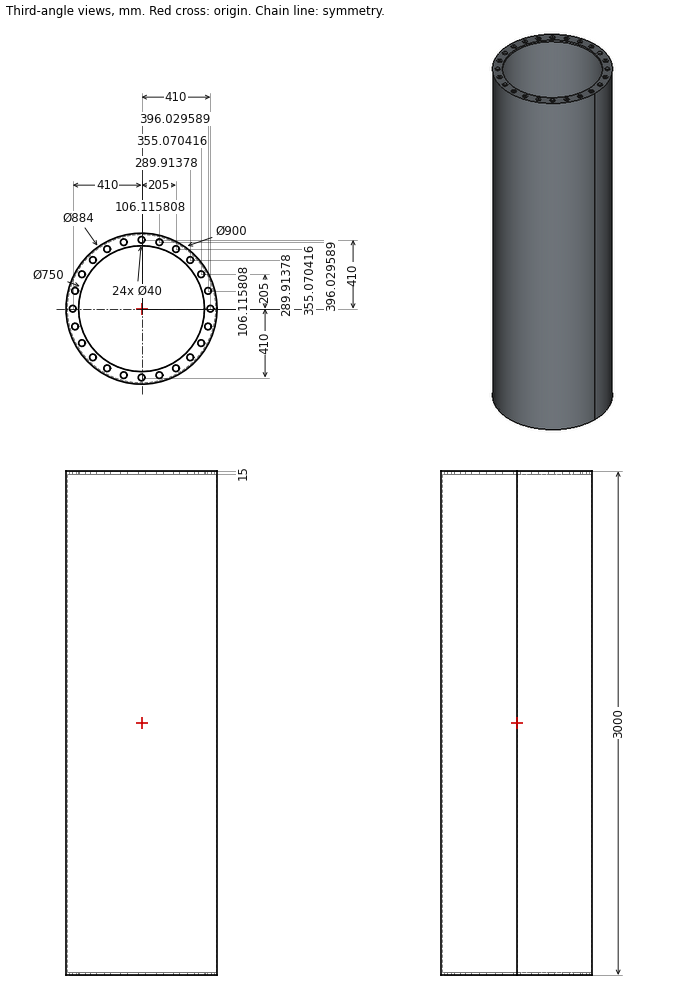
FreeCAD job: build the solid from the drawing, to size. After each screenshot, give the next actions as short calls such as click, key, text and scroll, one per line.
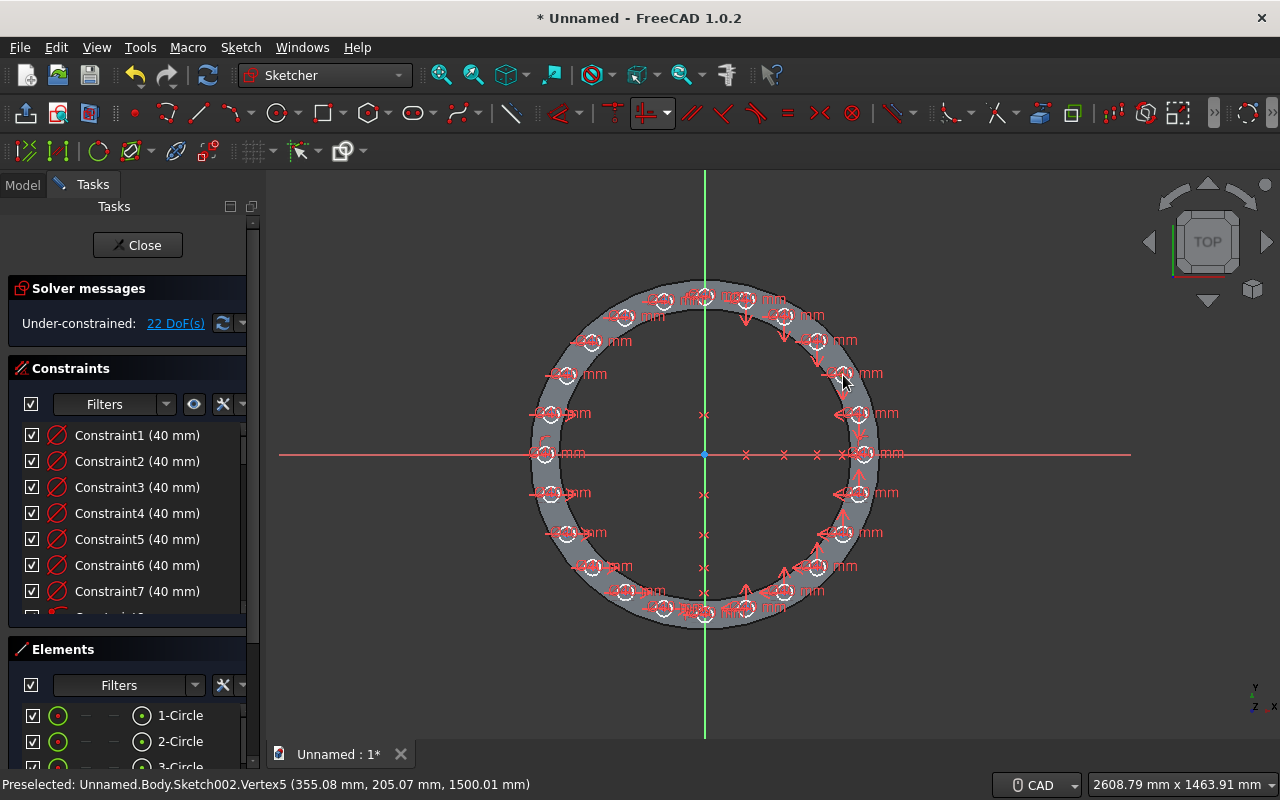
click(567, 376)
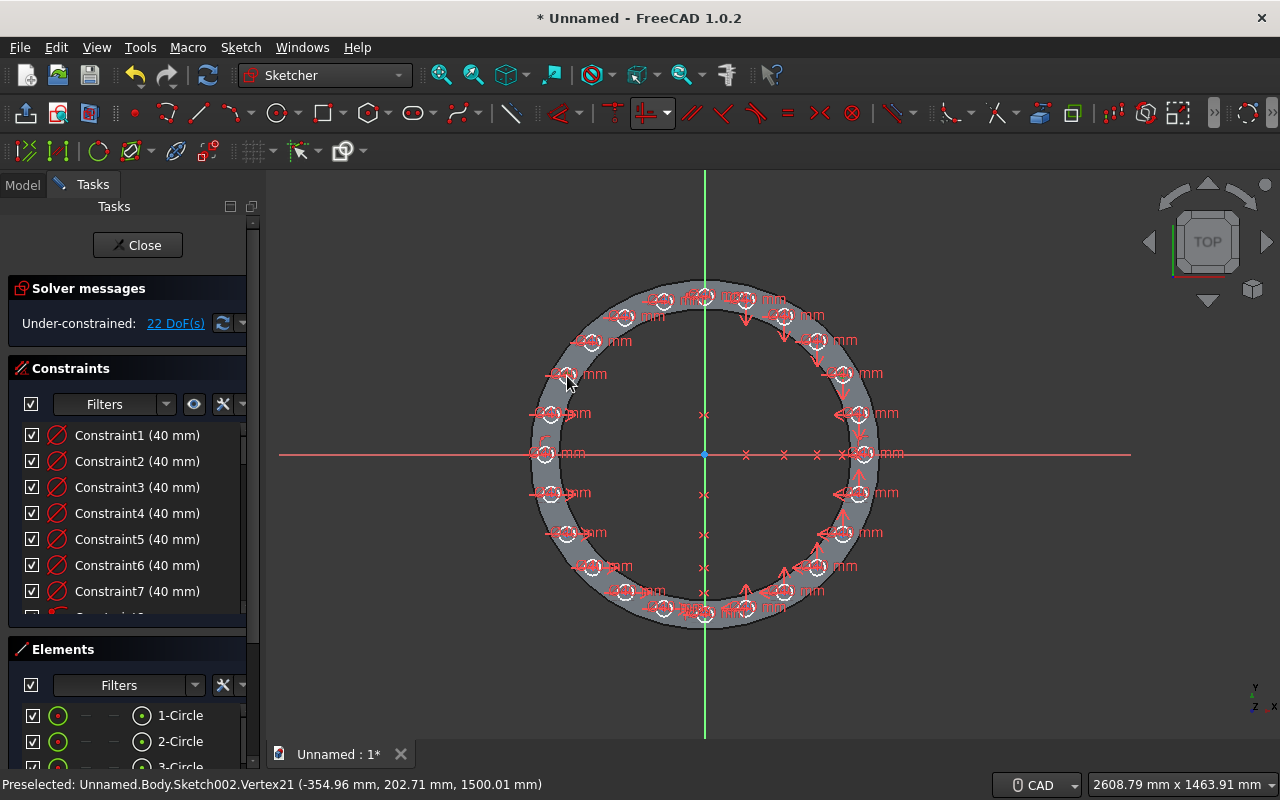
click(705, 674)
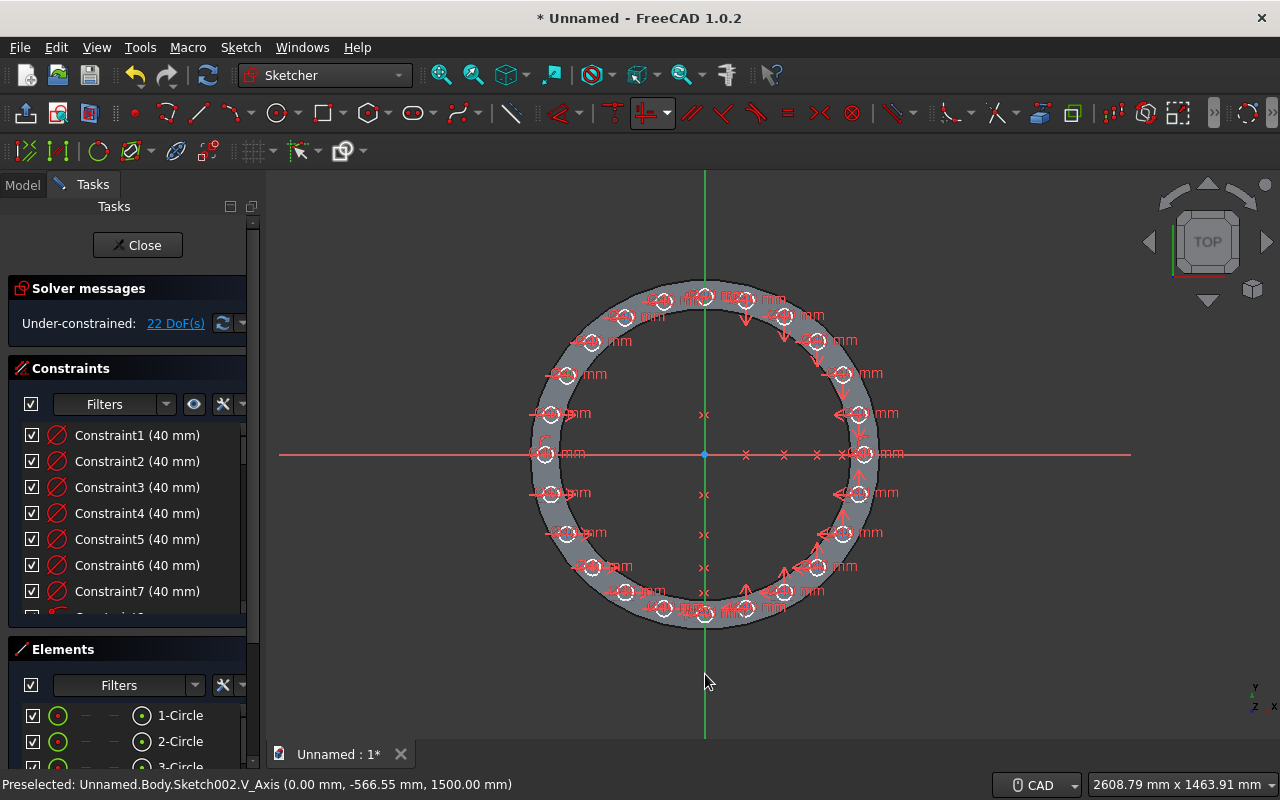
click(820, 114)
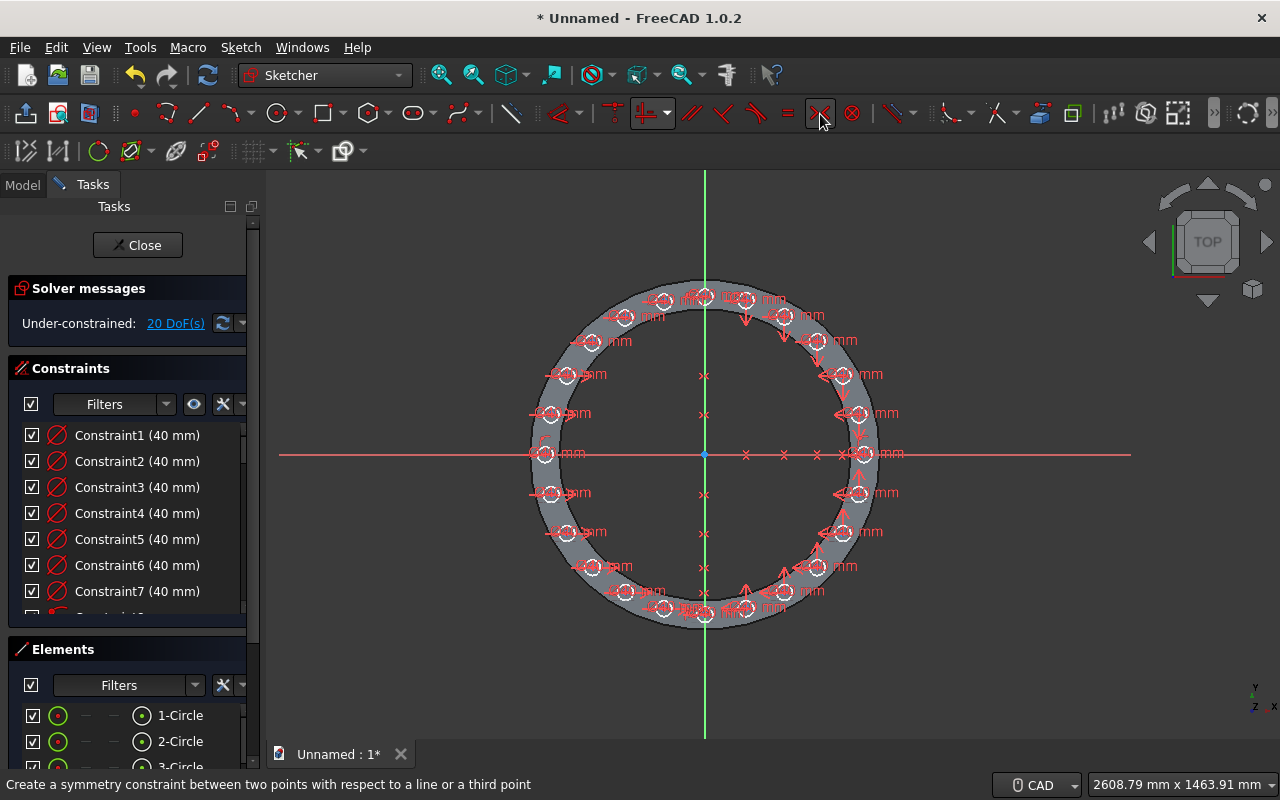
click(817, 342)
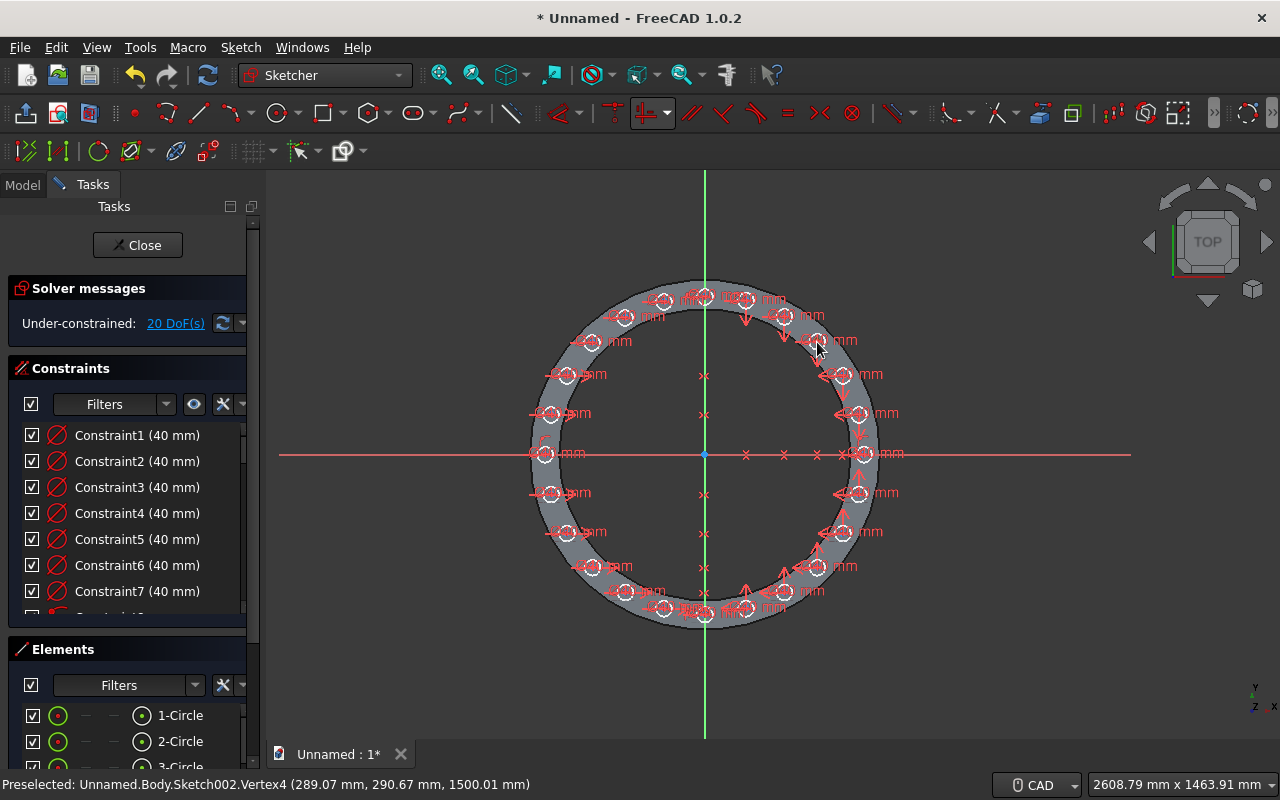
click(592, 343)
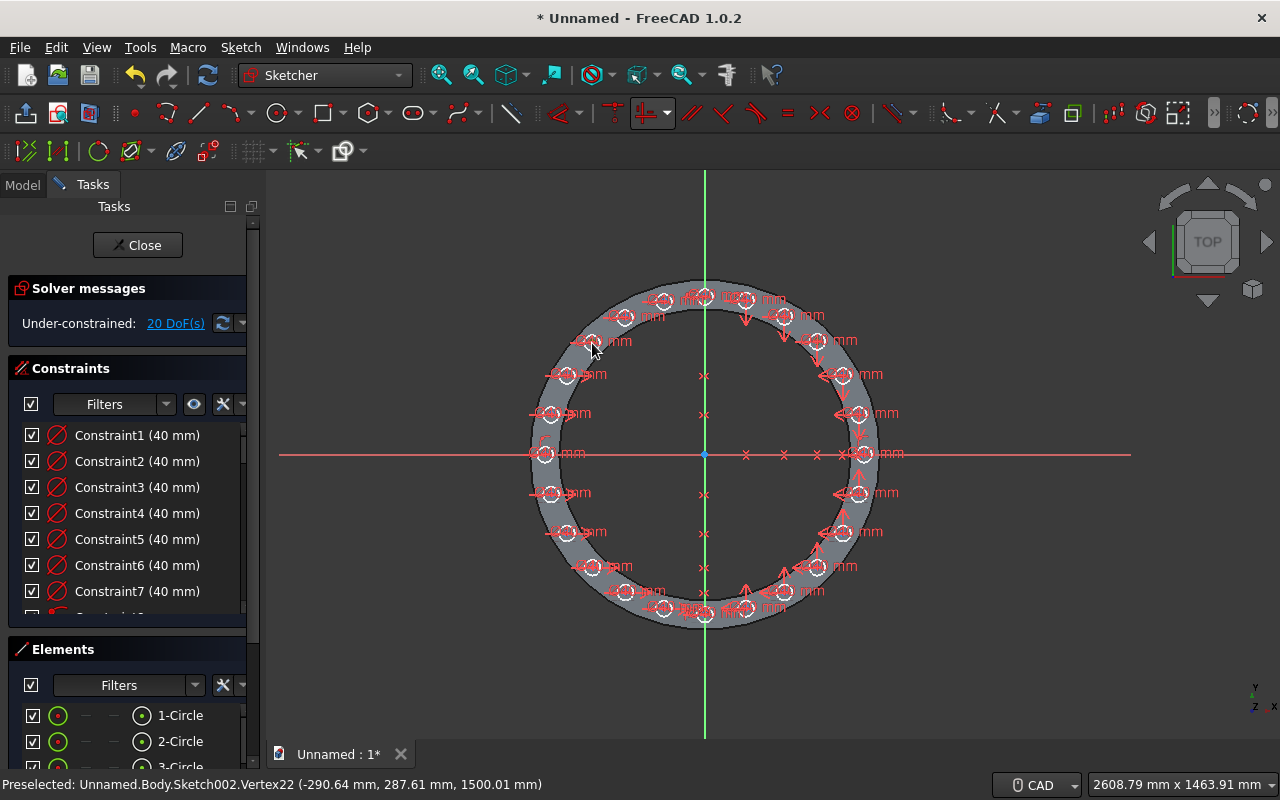
click(705, 674)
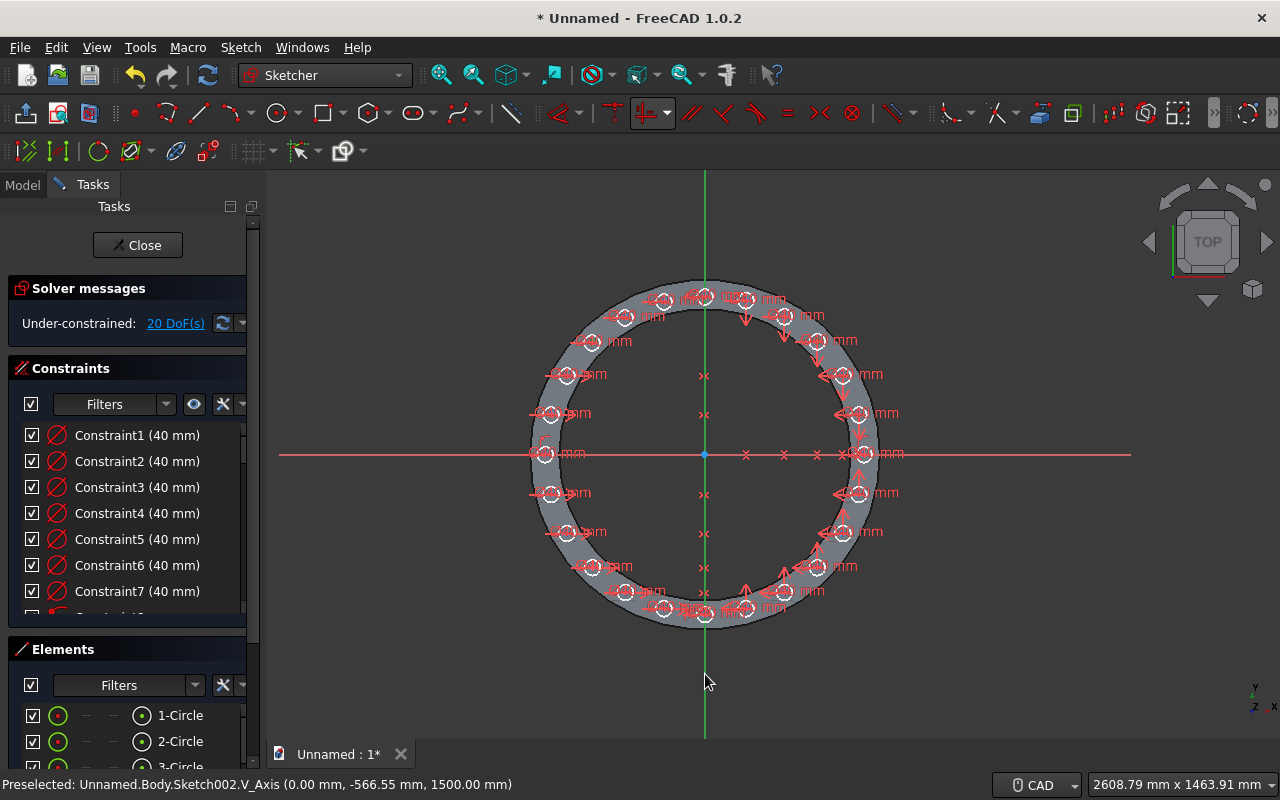
click(820, 114)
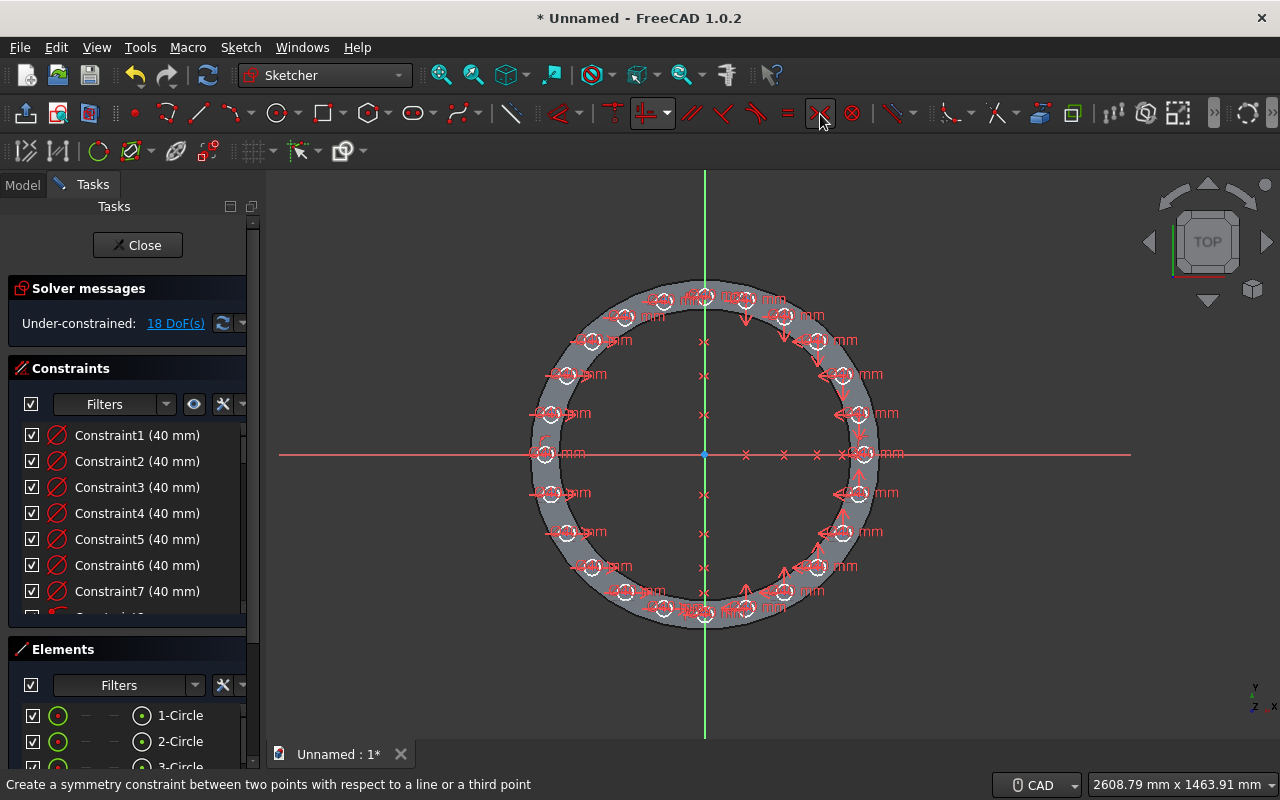
click(784, 317)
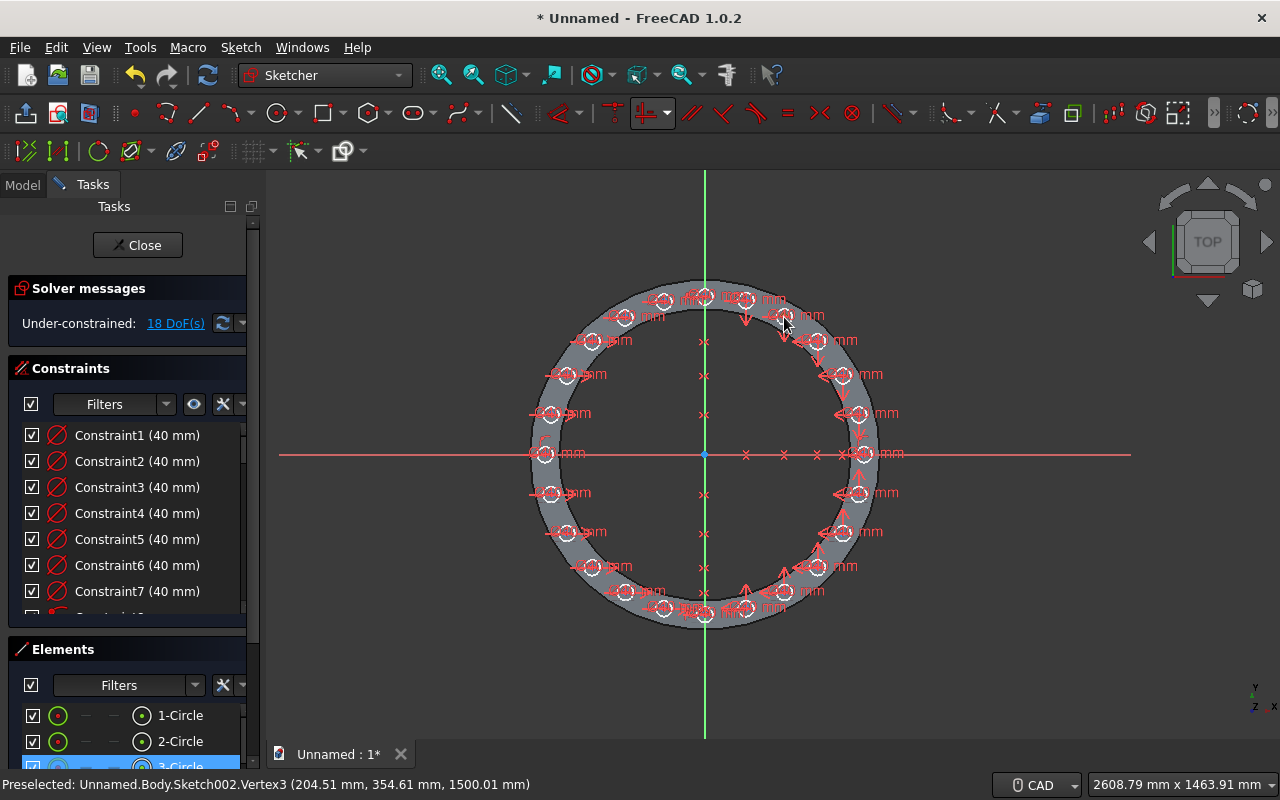
click(625, 318)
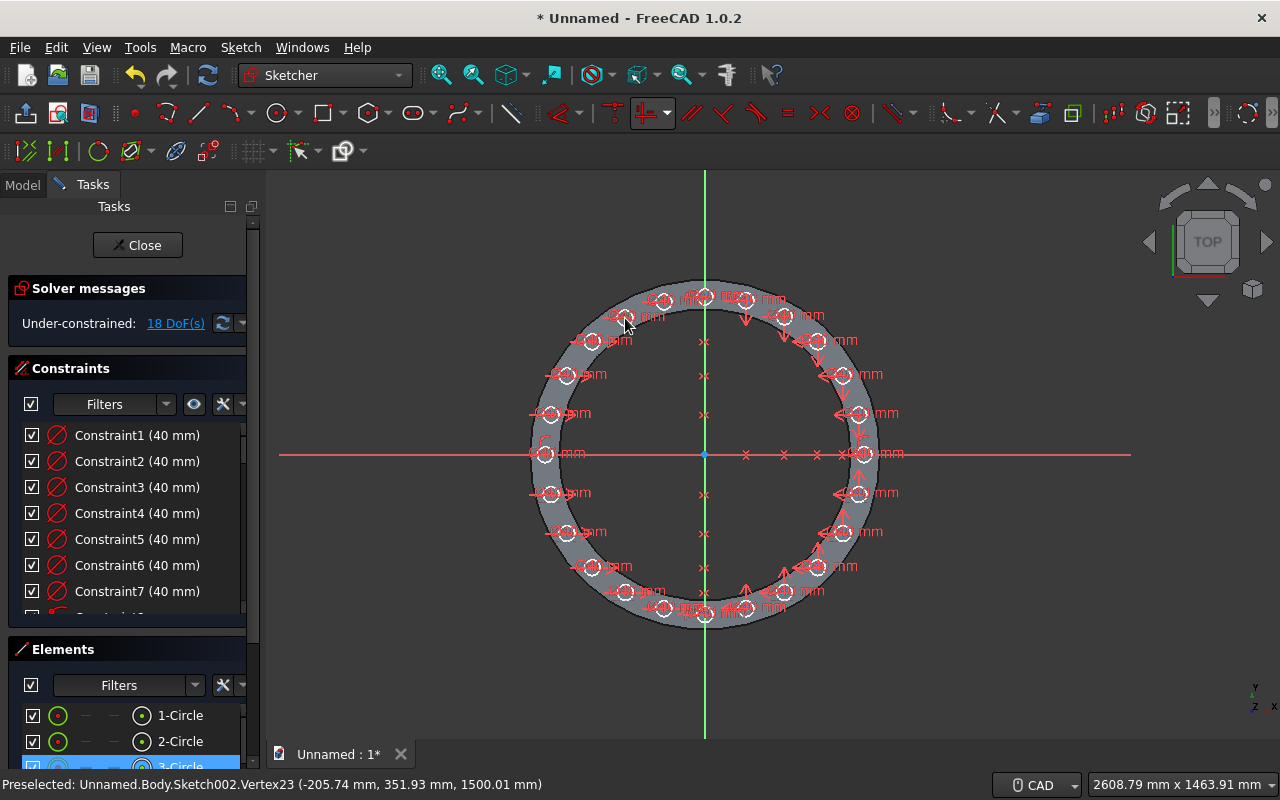
click(705, 674)